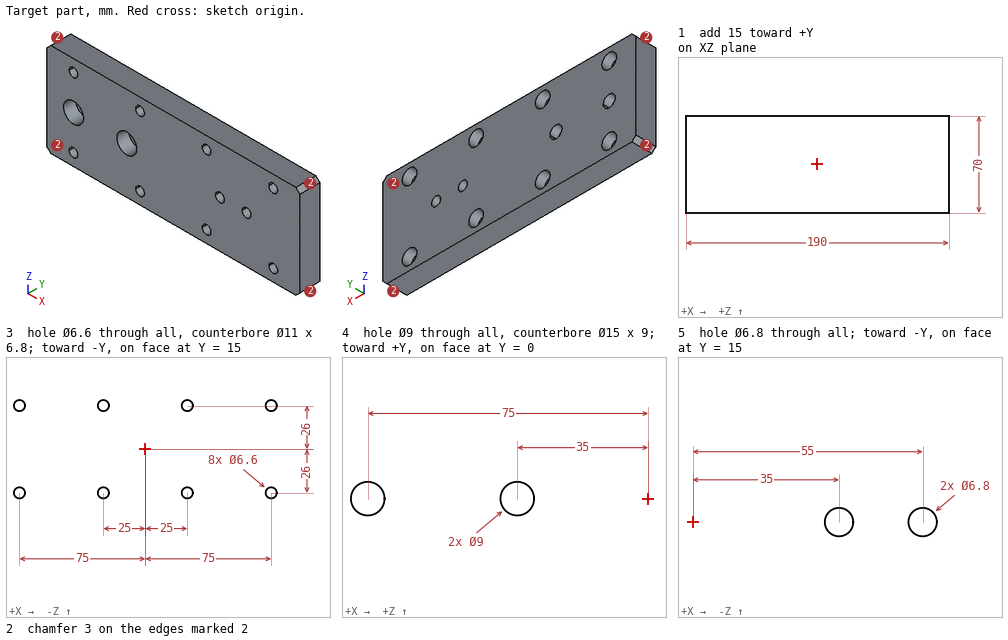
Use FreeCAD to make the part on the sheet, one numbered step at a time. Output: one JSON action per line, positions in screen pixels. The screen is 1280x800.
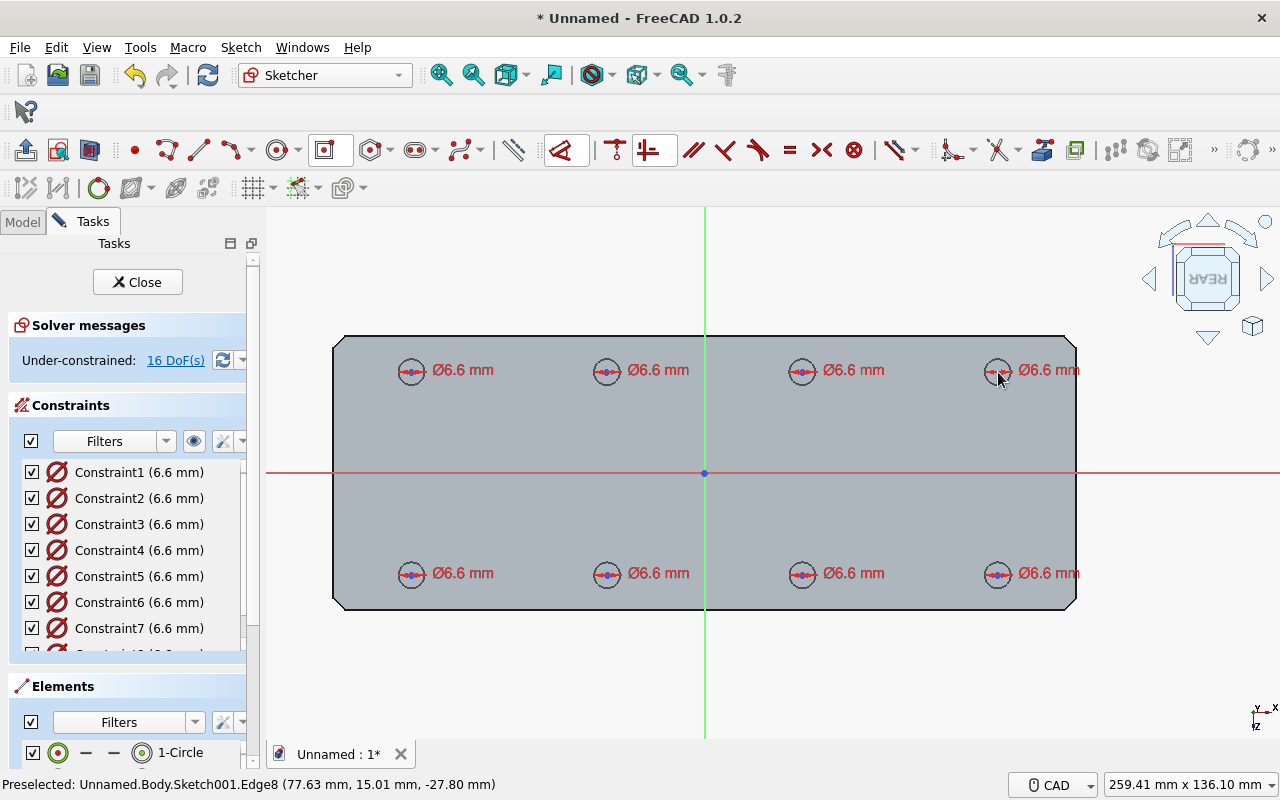
{"action": "left_click", "coordinate": [998, 575]}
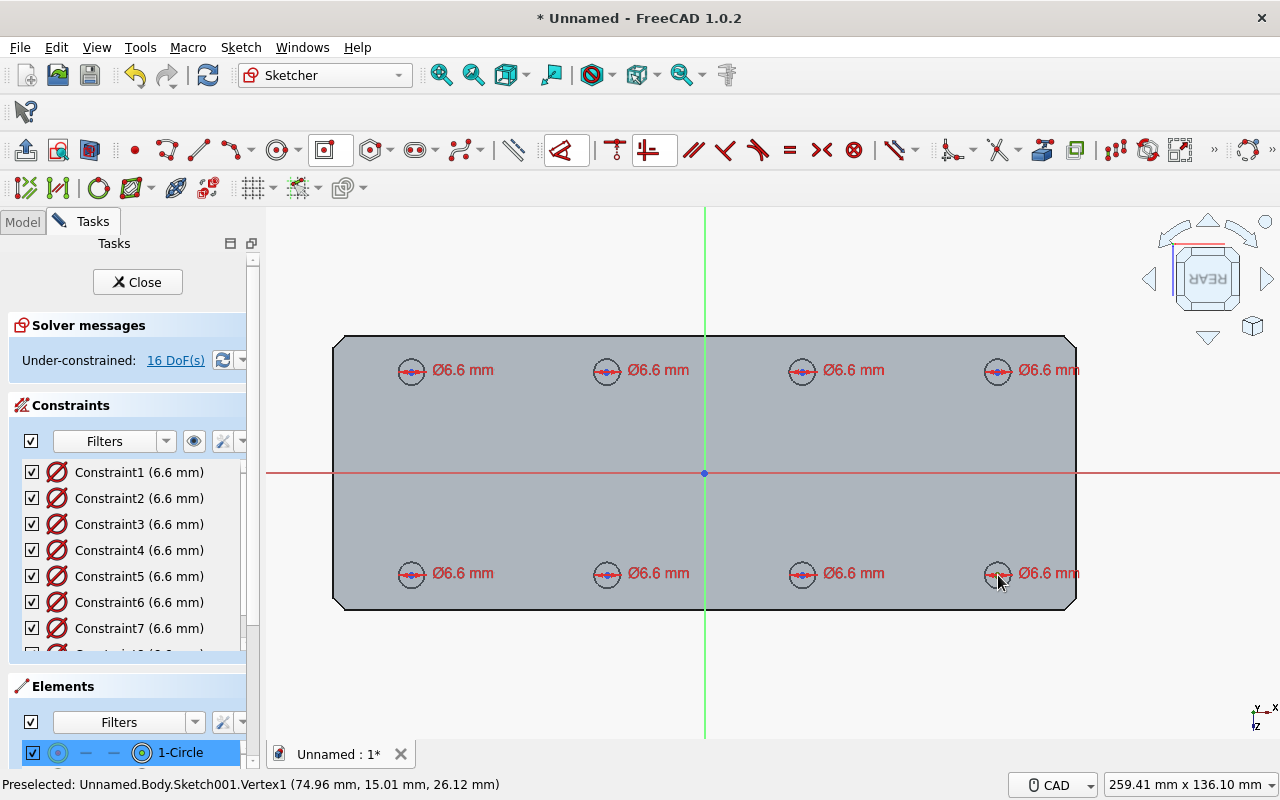
{"action": "left_click", "coordinate": [802, 575]}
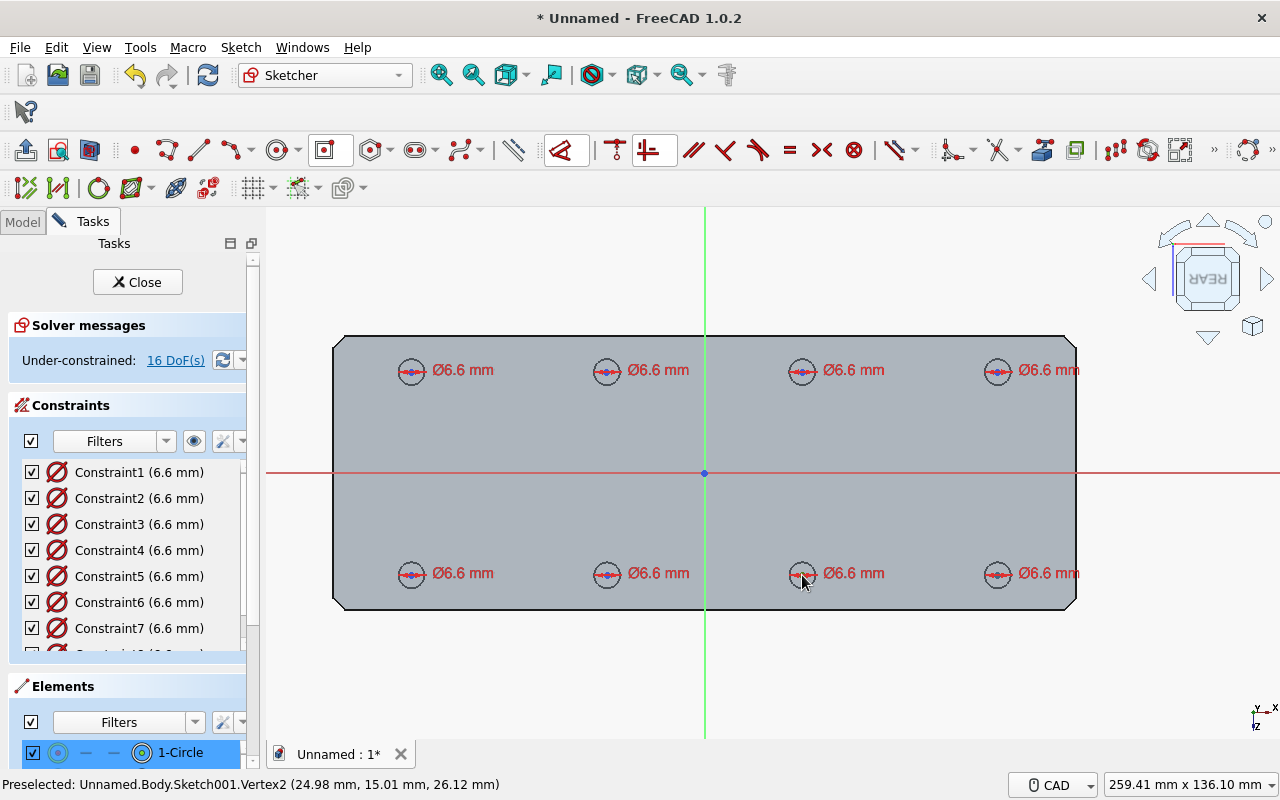
{"action": "left_click", "coordinate": [672, 150]}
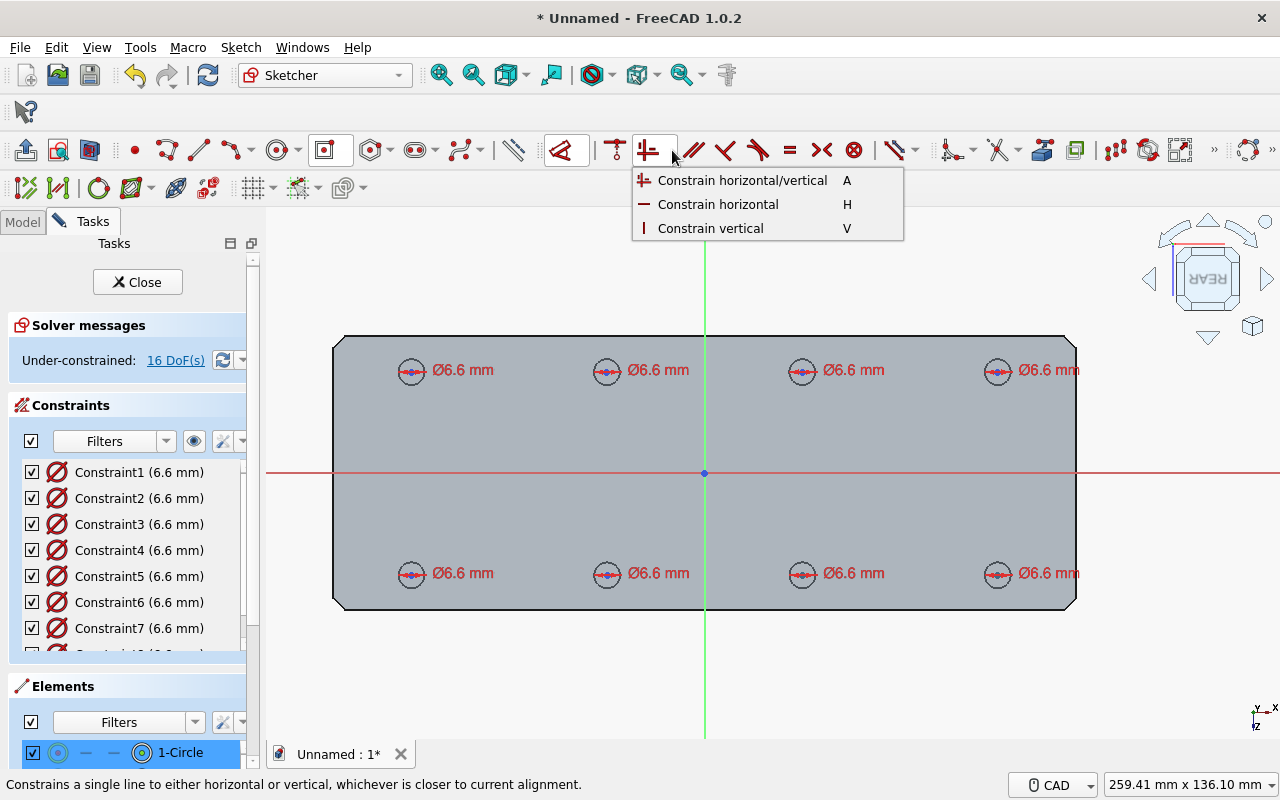
{"action": "left_click", "coordinate": [768, 204]}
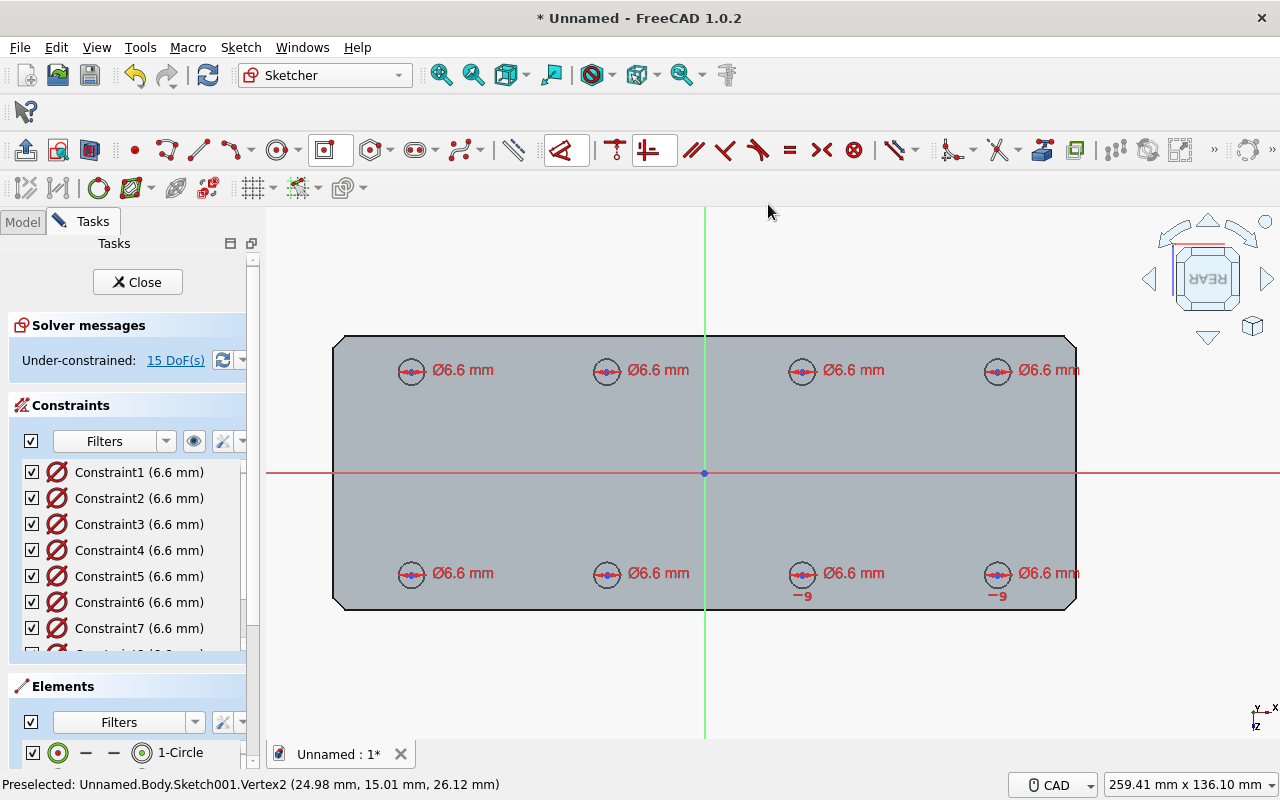
{"action": "left_click", "coordinate": [802, 575]}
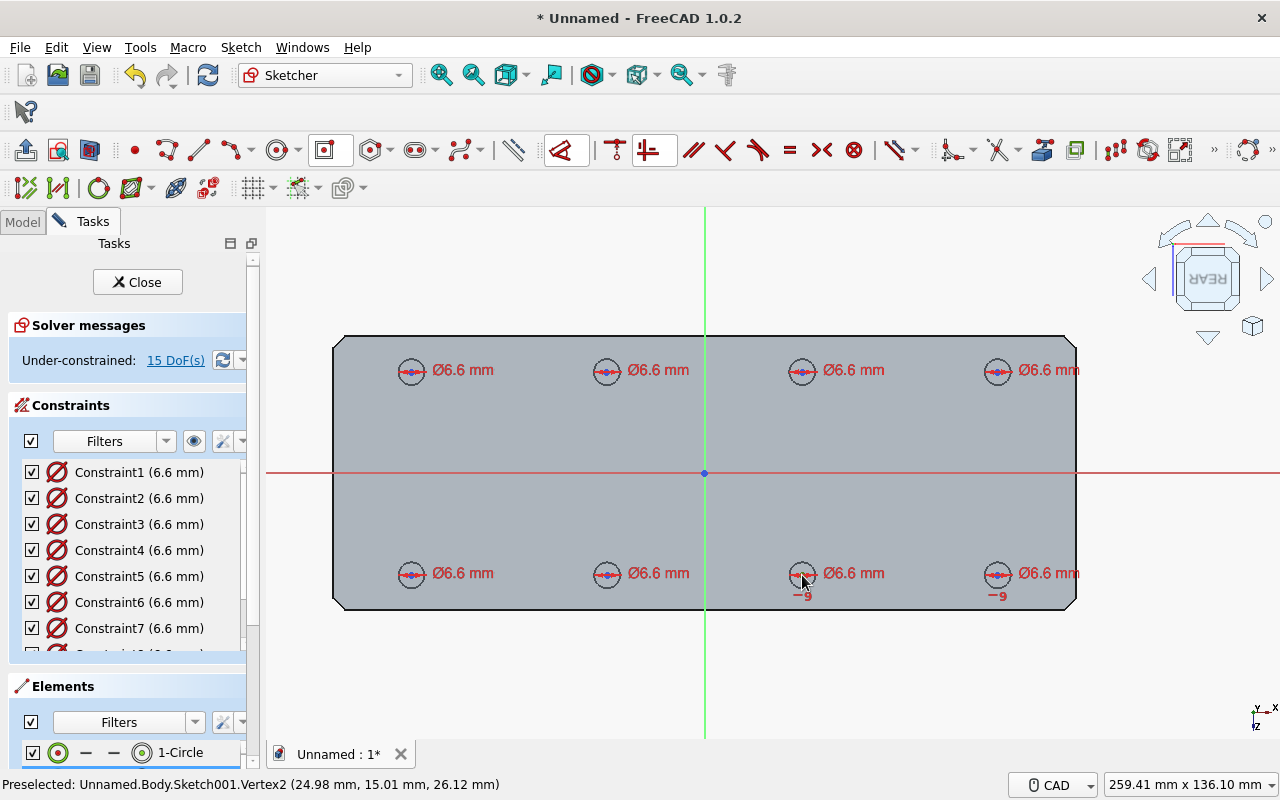
{"action": "left_click", "coordinate": [607, 575]}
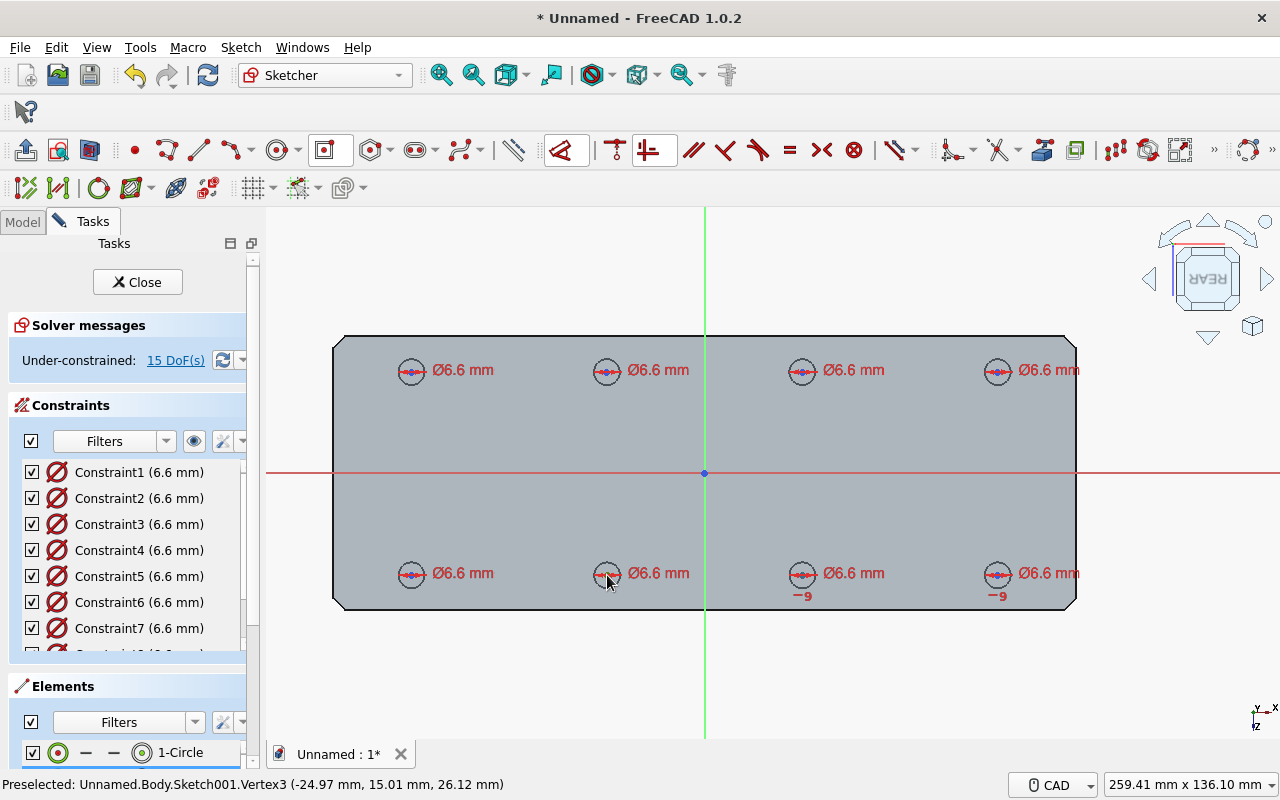
{"action": "key", "text": "h"}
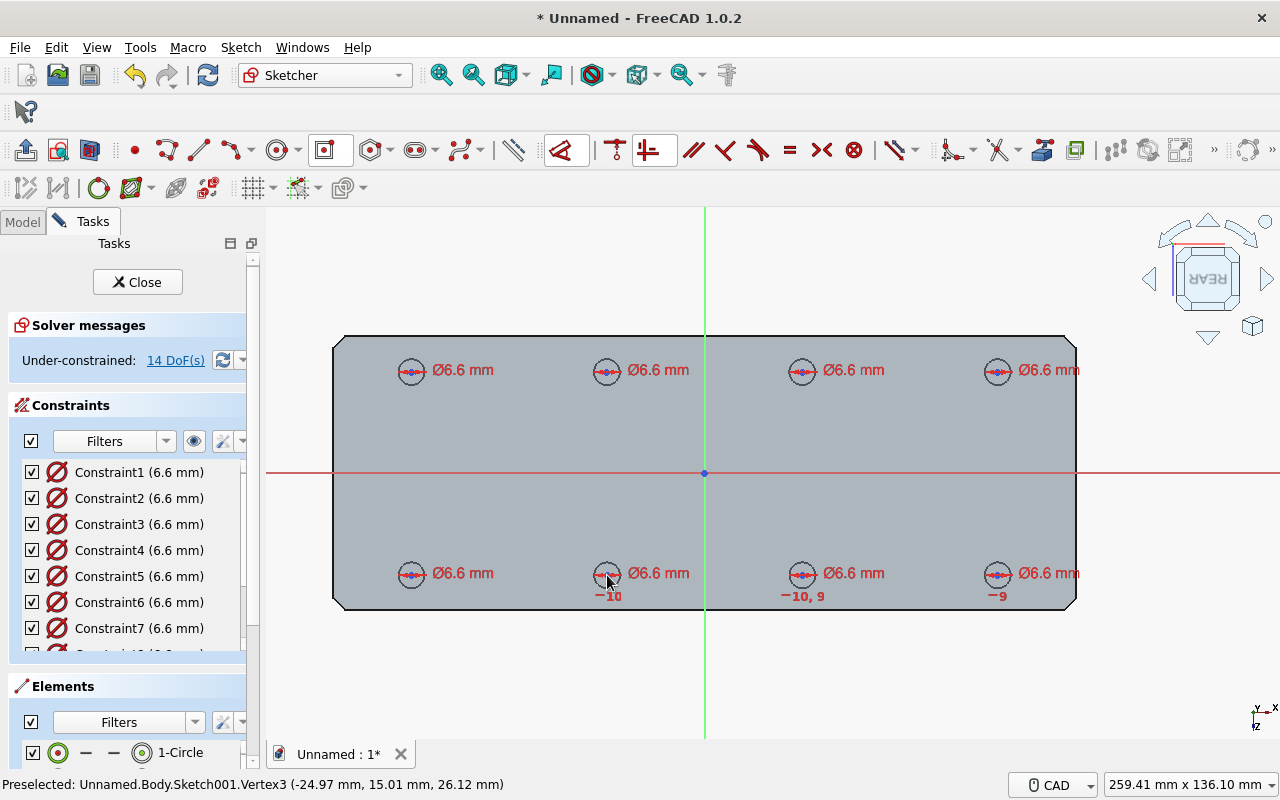
{"action": "left_click", "coordinate": [607, 575]}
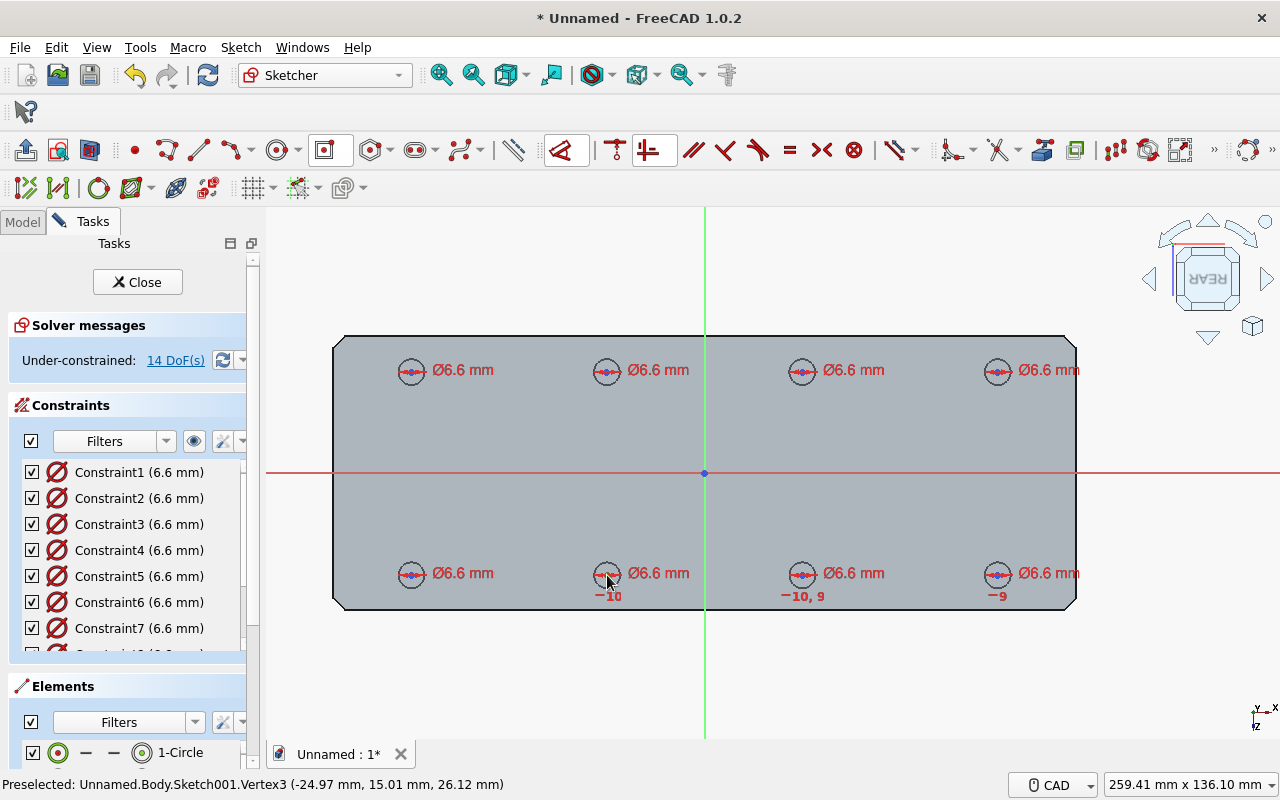
{"action": "left_click", "coordinate": [412, 575]}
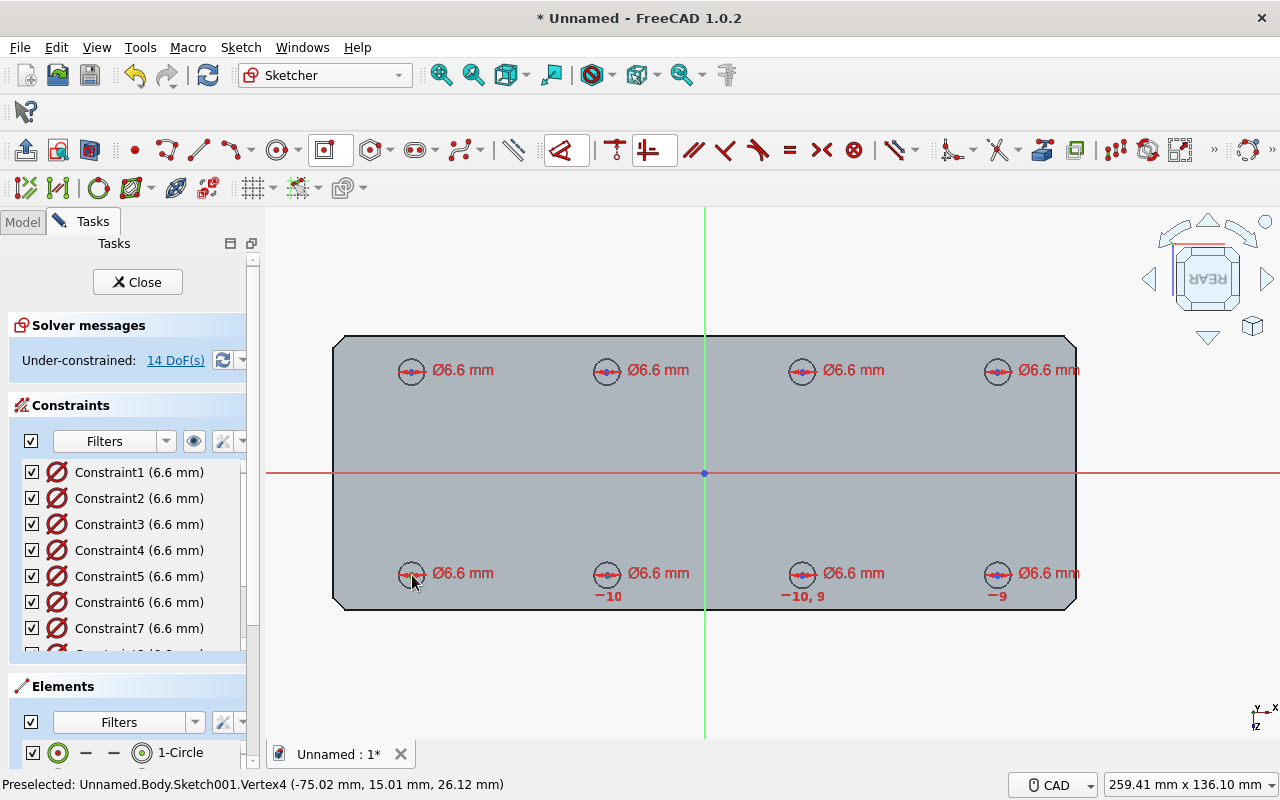
{"action": "key", "text": "h"}